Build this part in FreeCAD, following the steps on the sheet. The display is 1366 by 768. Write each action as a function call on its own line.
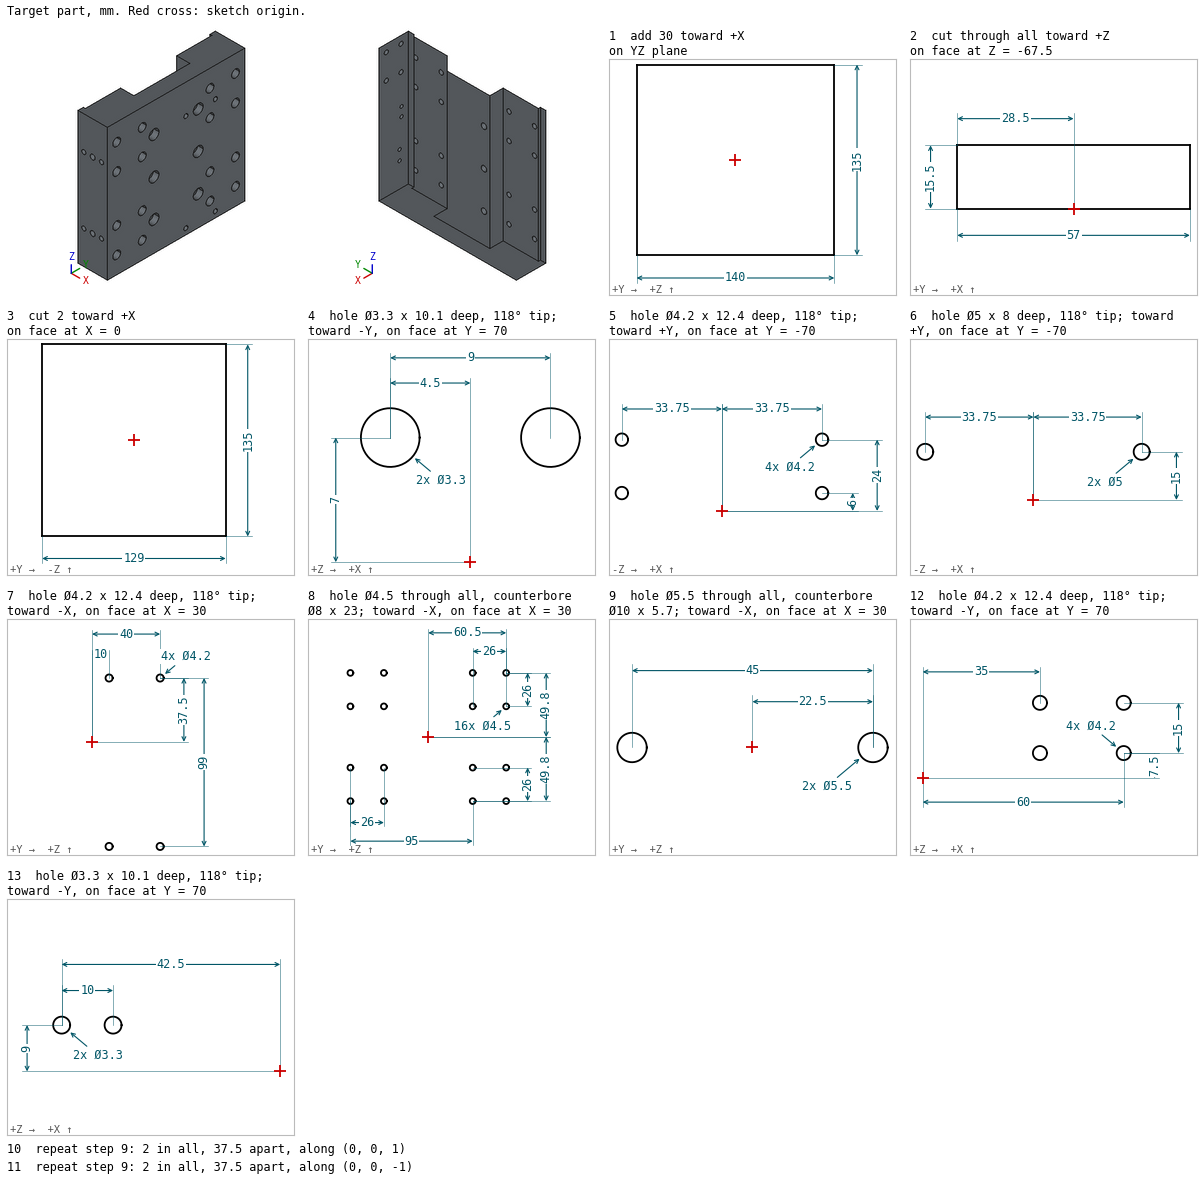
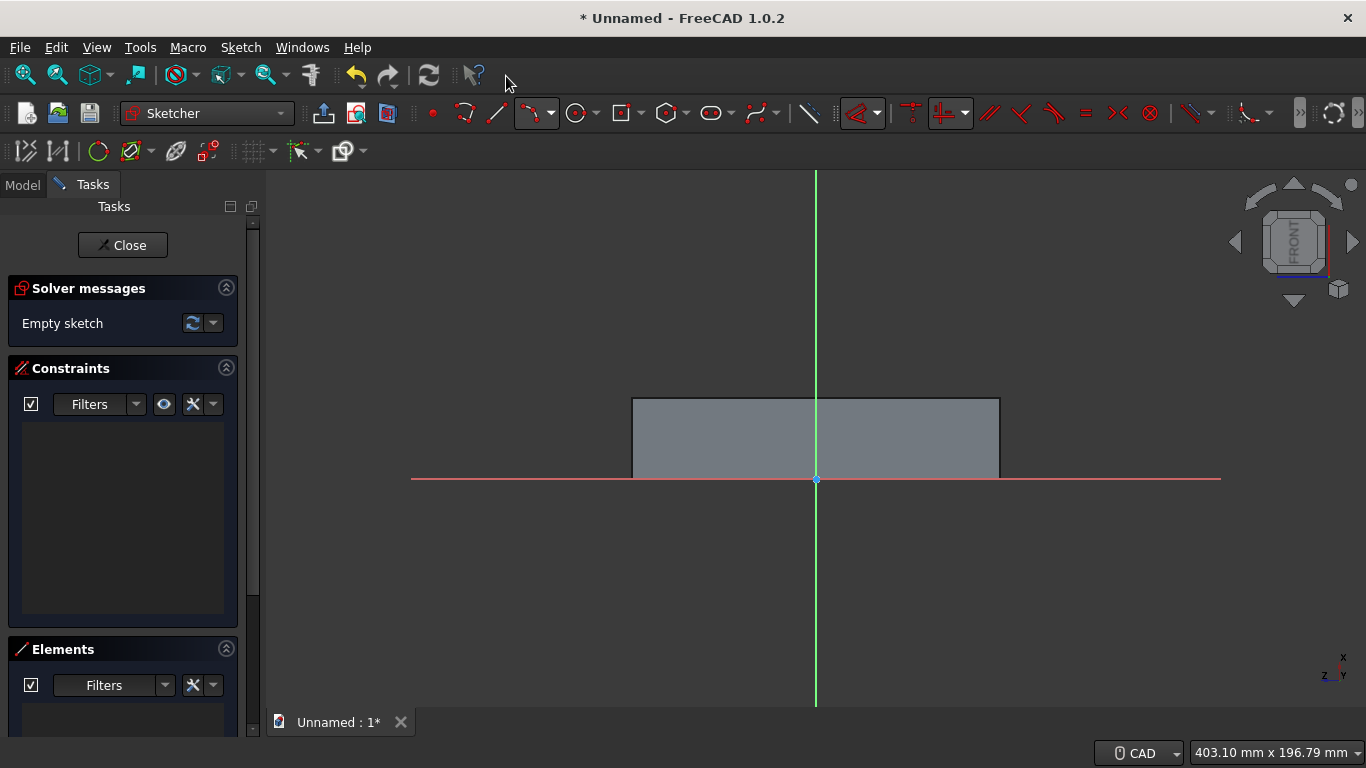
scroll(846, 446, up, 6)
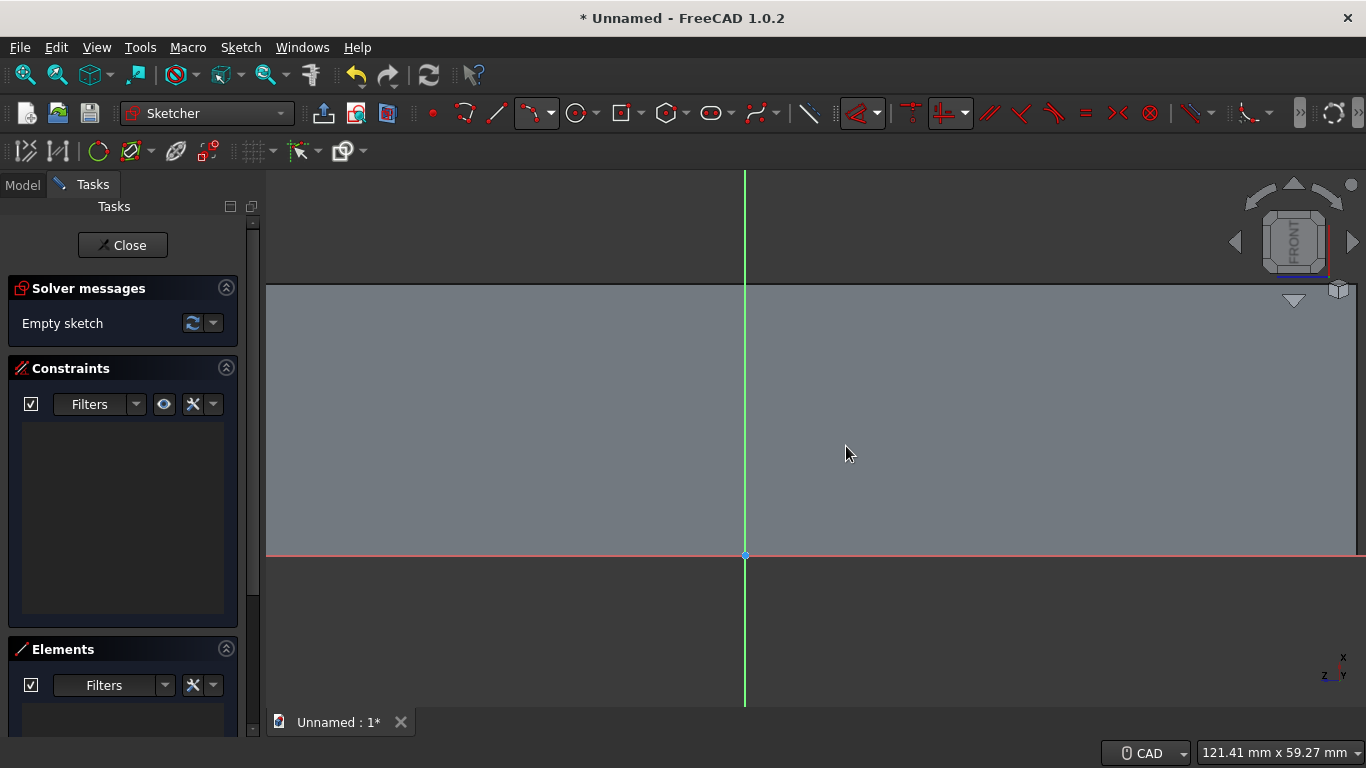
click(576, 114)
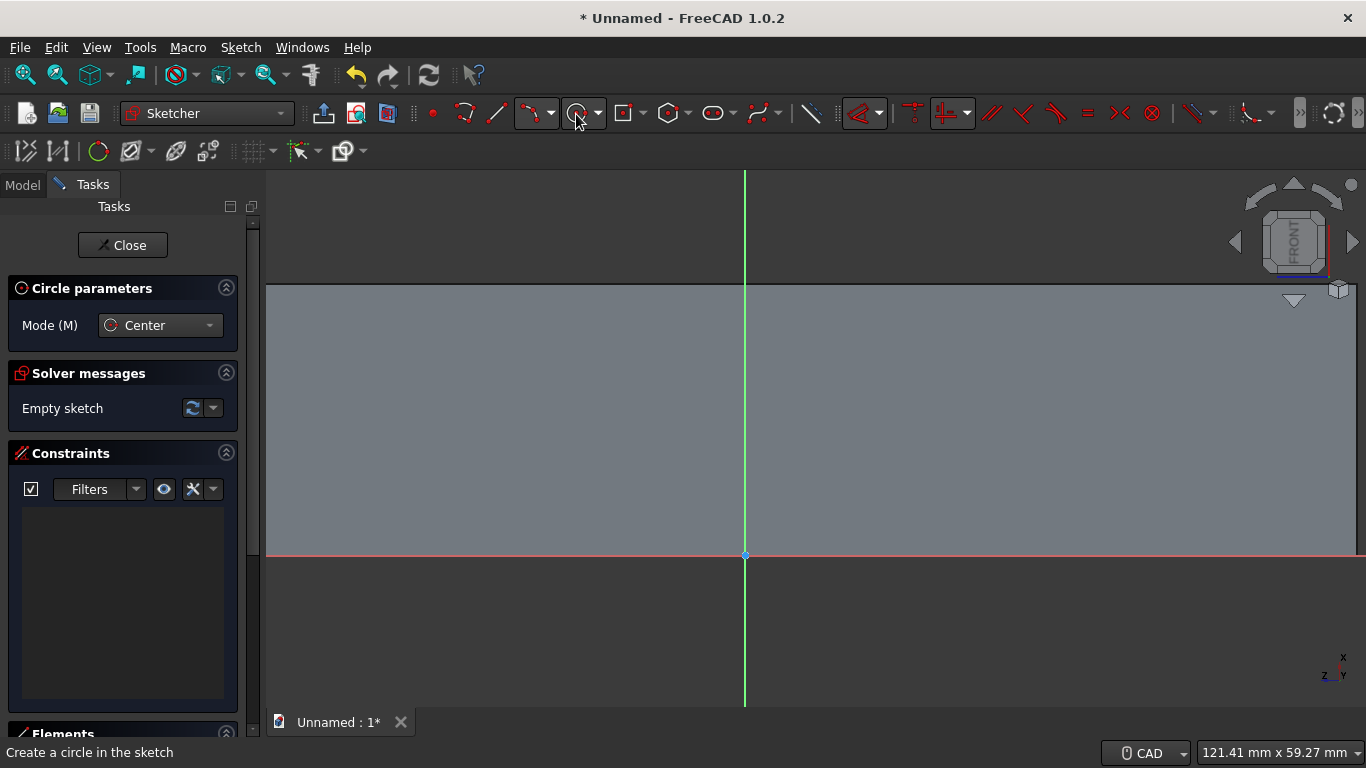
click(1051, 338)
click(1064, 325)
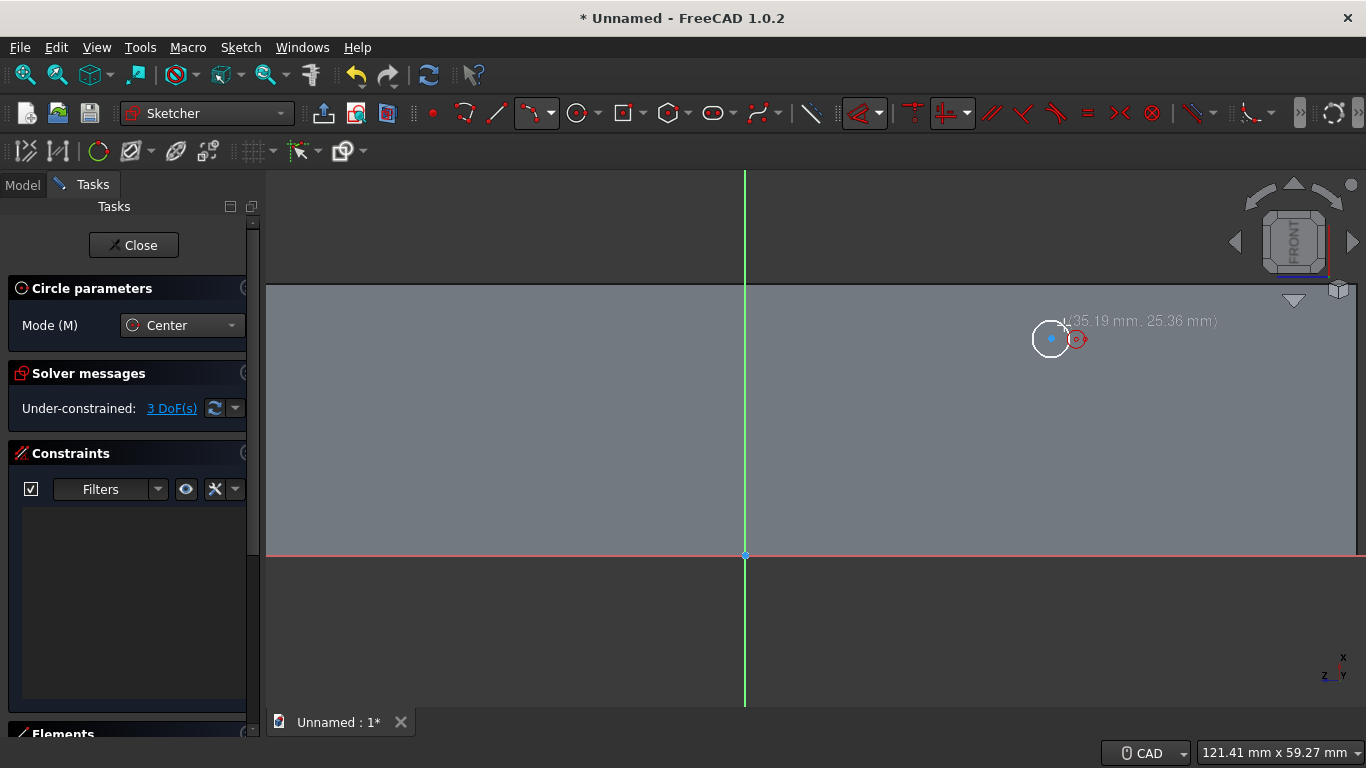
click(1051, 501)
click(1064, 488)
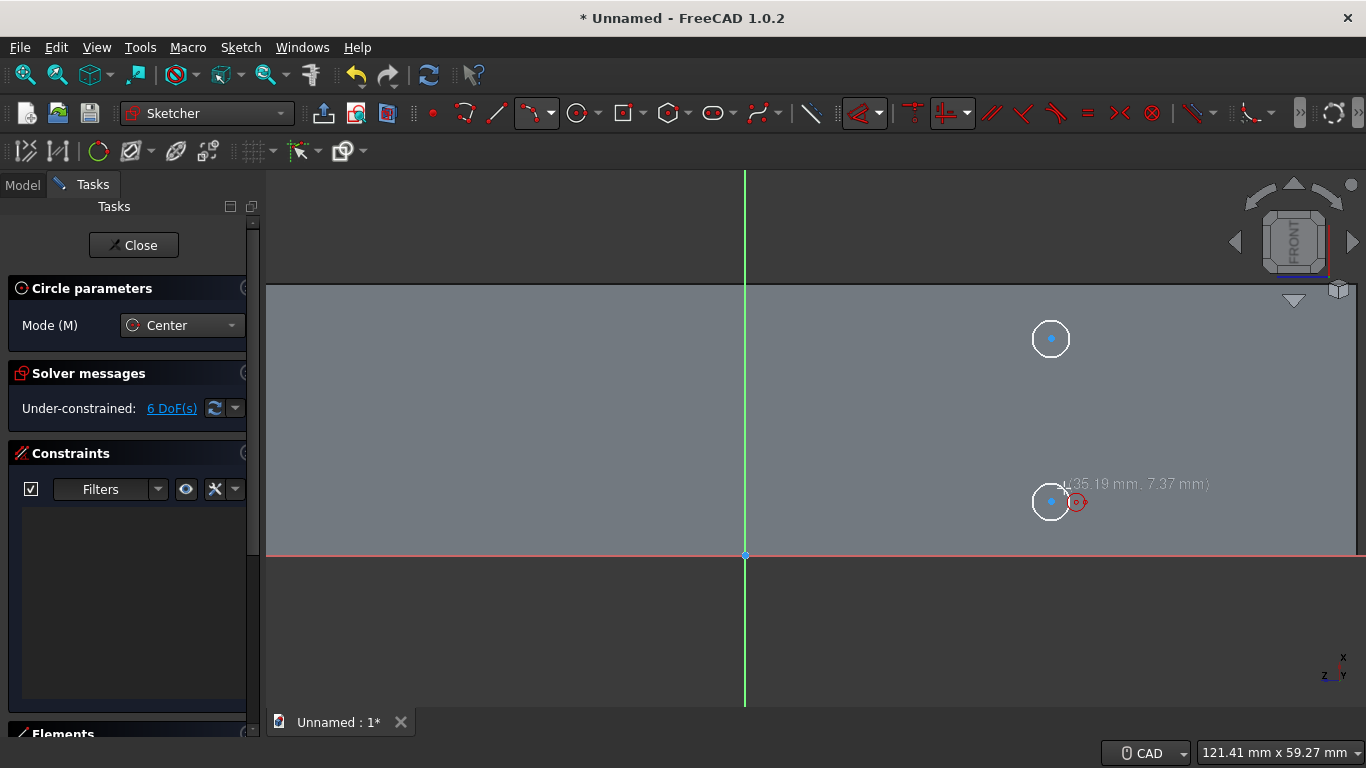
click(439, 338)
click(453, 325)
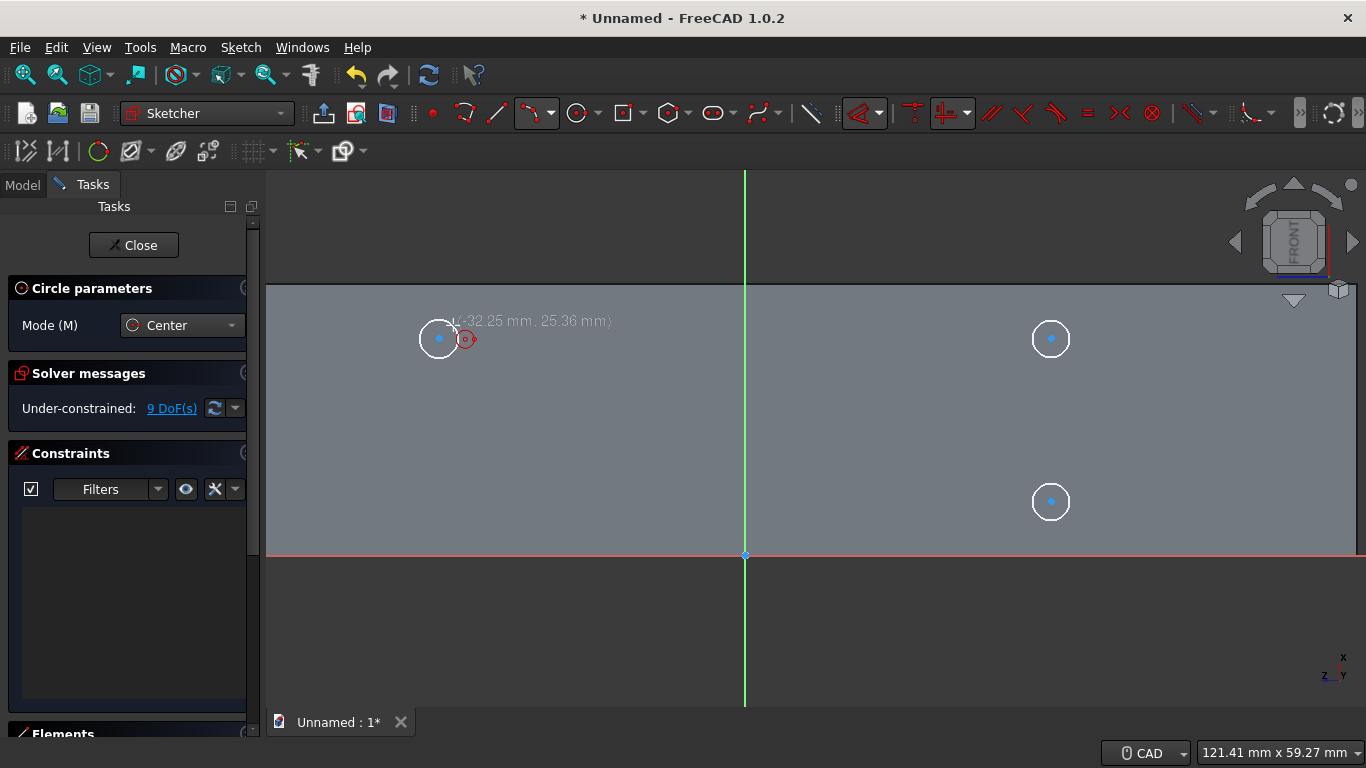
click(439, 501)
click(453, 488)
key(Escape)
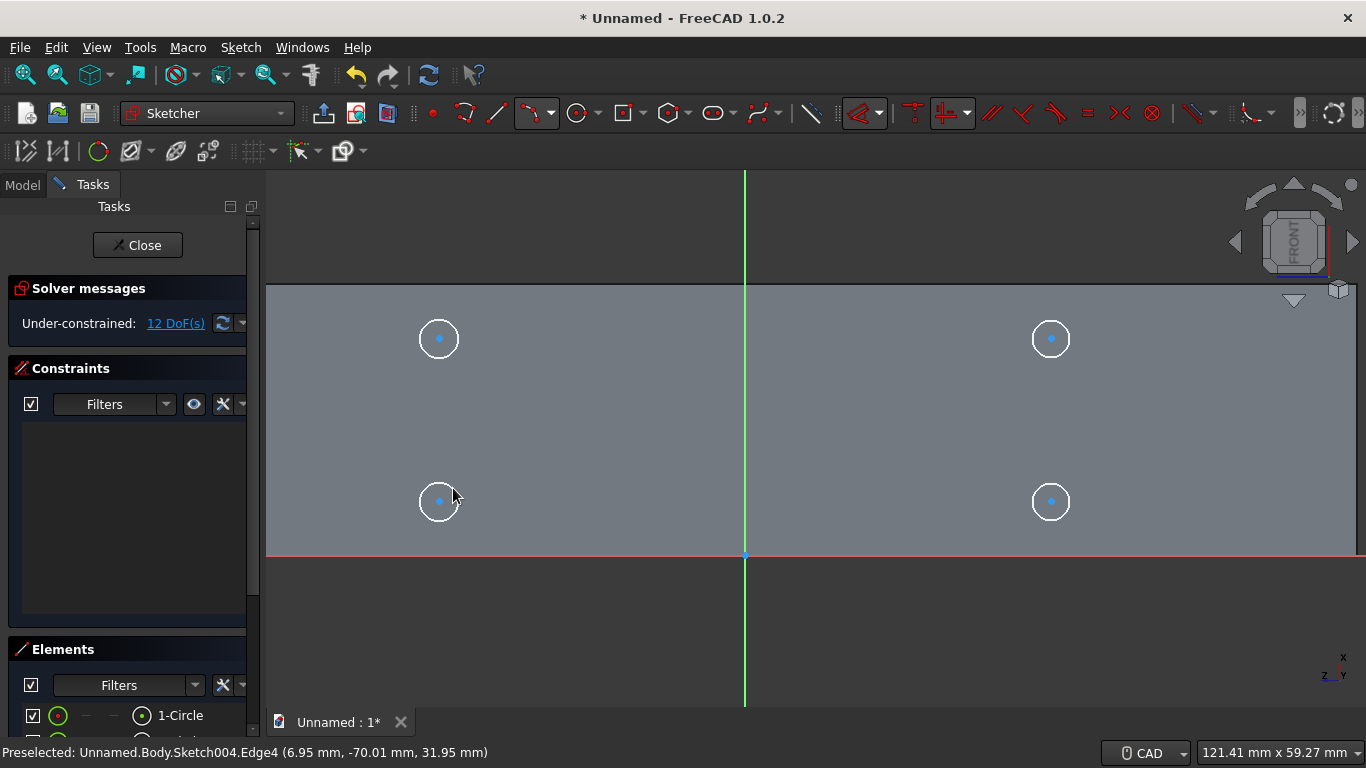
click(1064, 326)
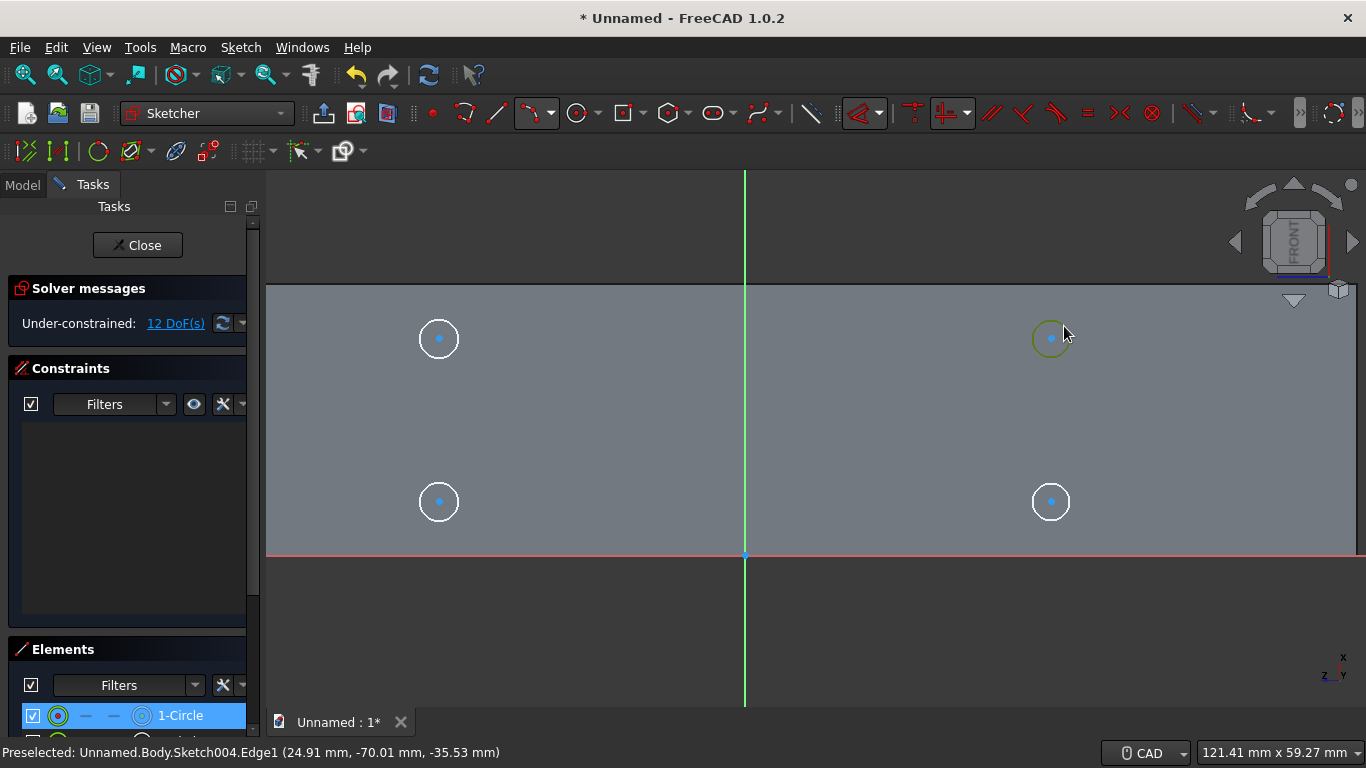
click(1064, 489)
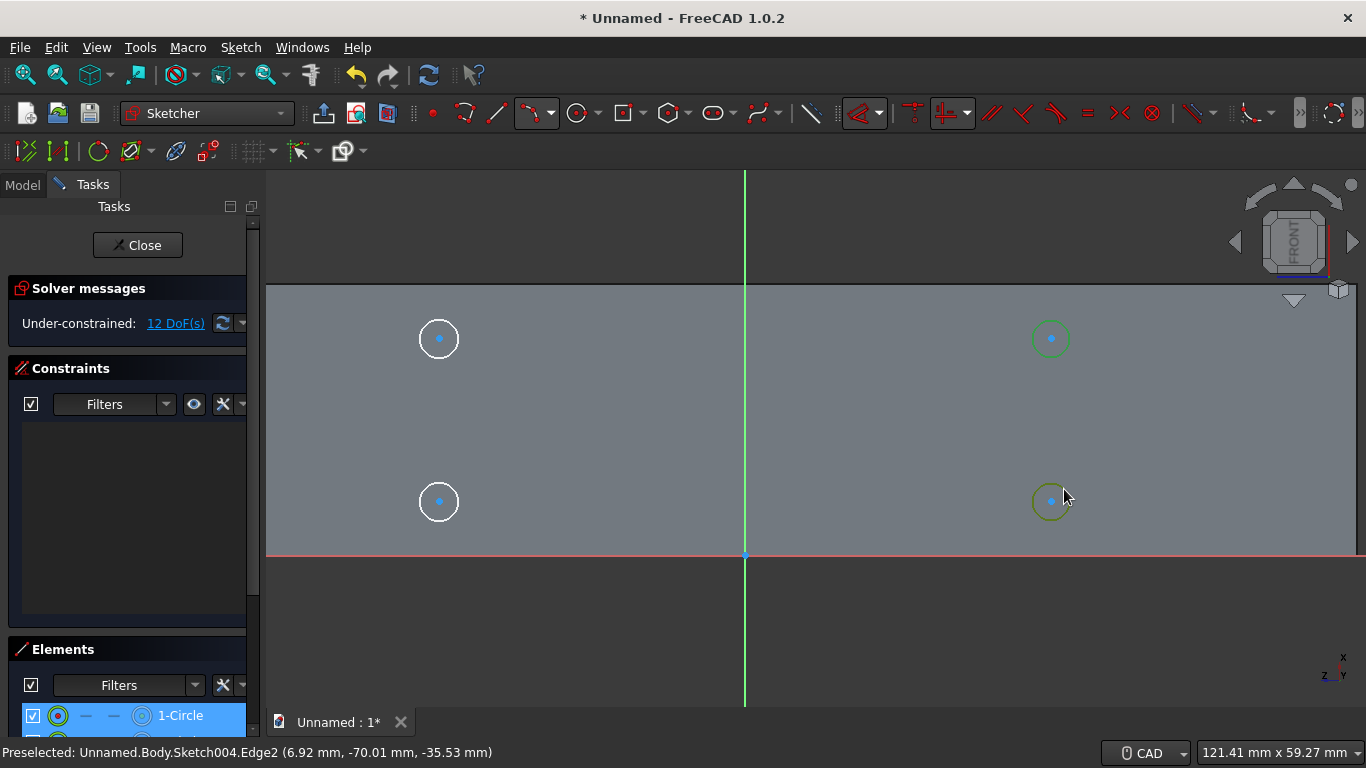
click(452, 325)